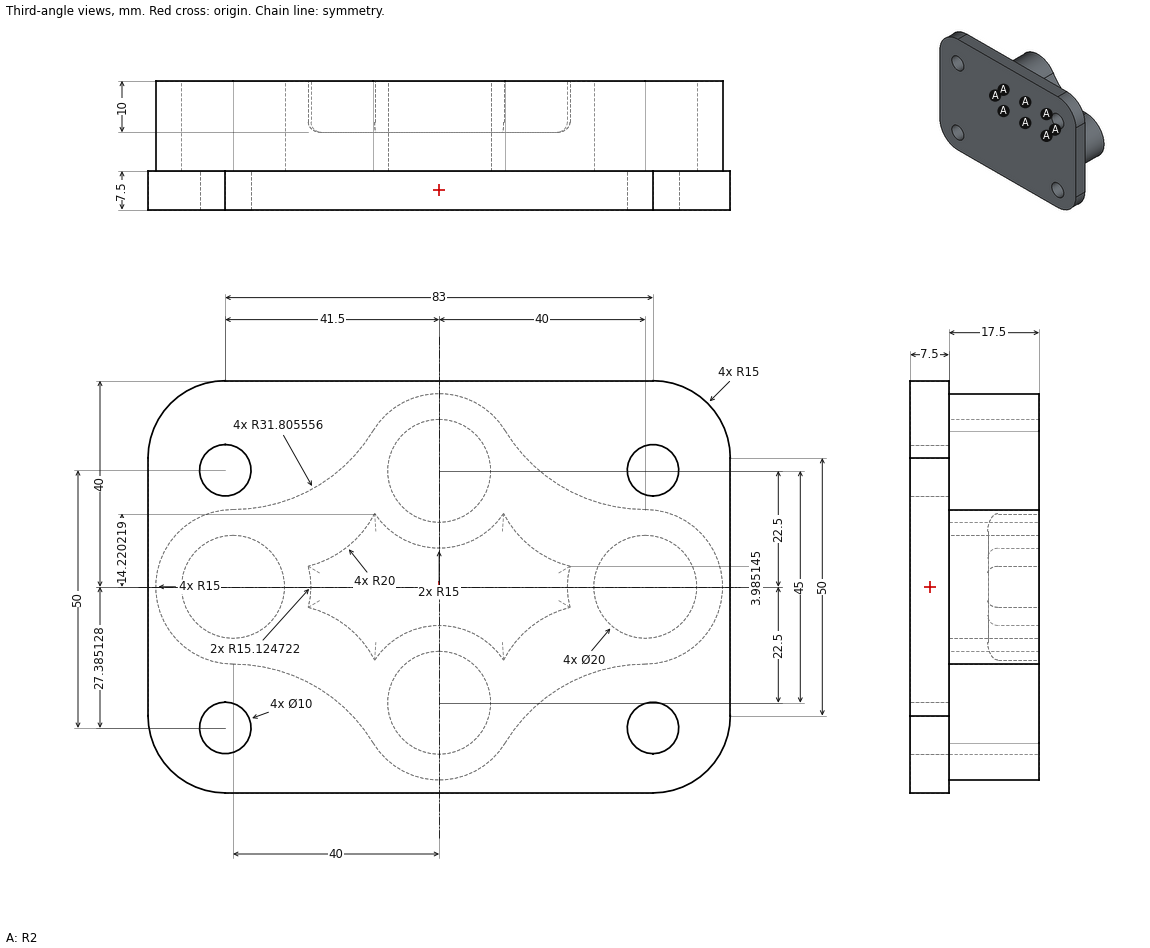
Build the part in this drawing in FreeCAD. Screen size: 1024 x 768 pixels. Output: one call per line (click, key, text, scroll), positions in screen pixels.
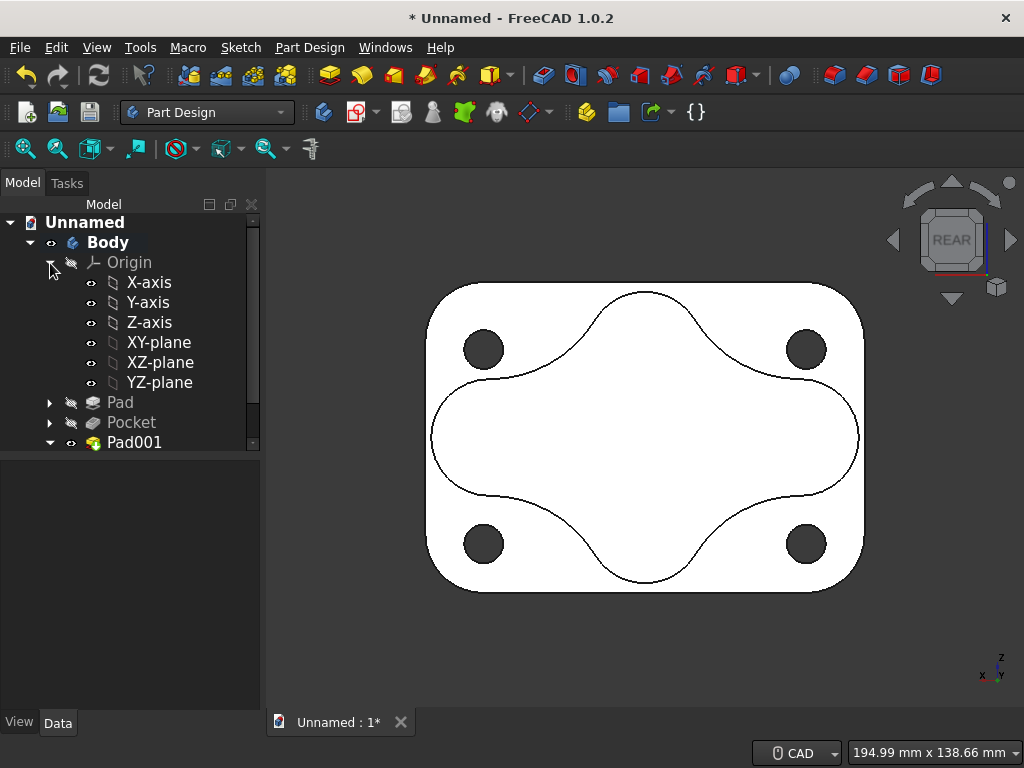
click(136, 363)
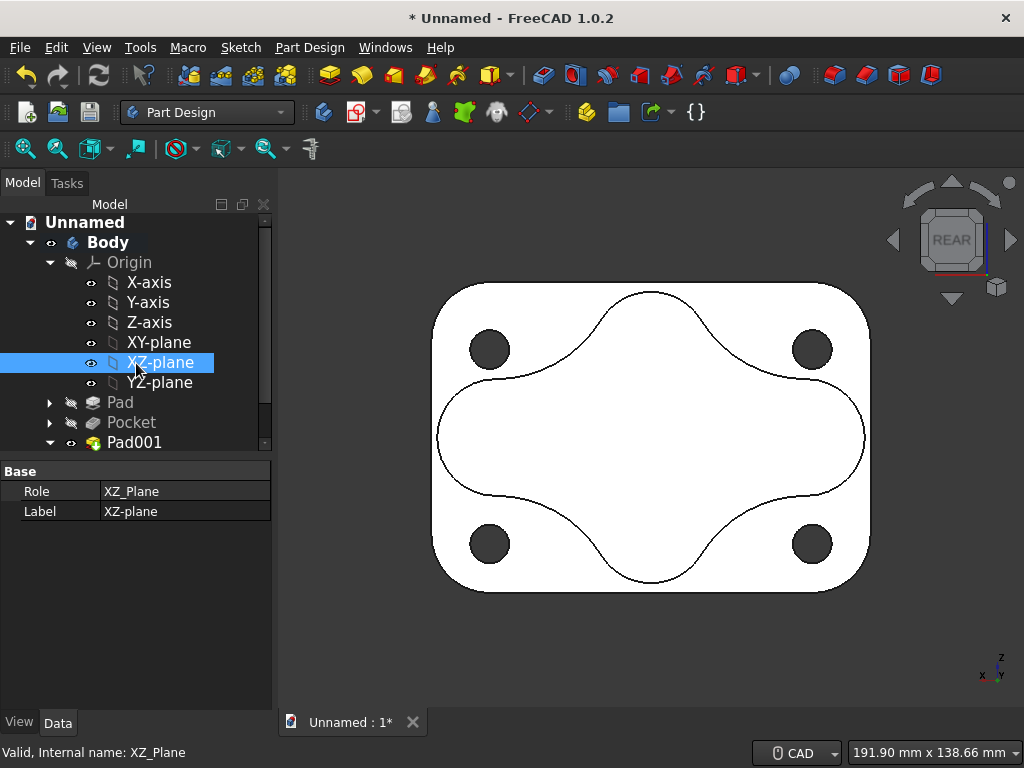
click(530, 112)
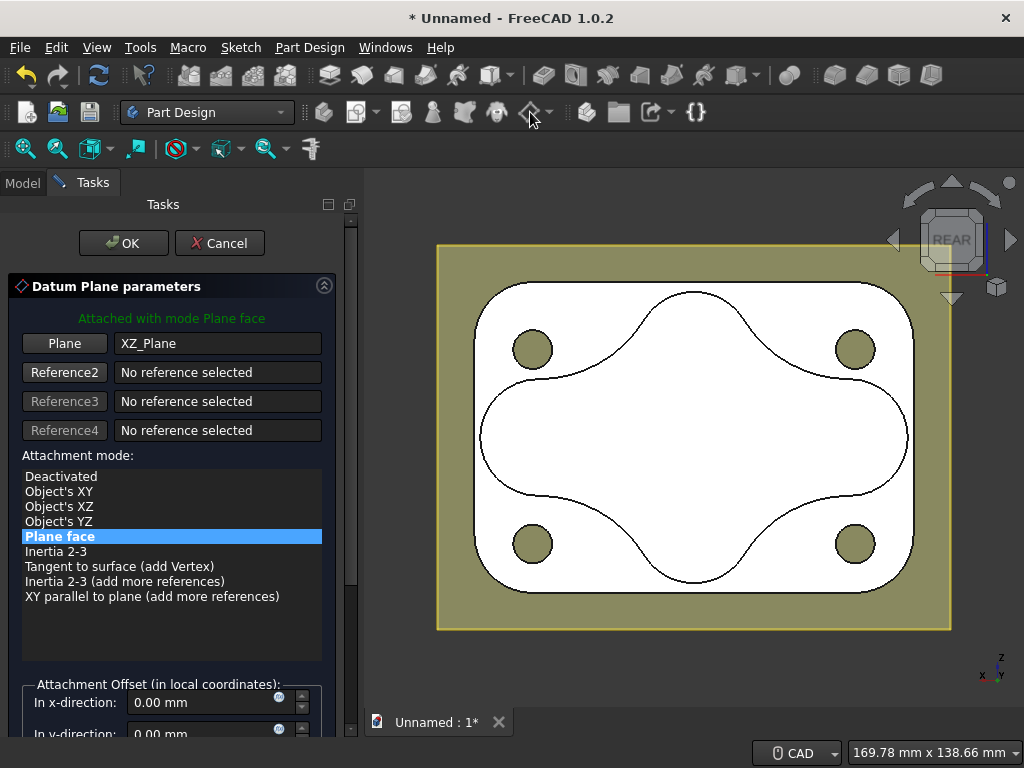
scroll(351, 475, down, 2)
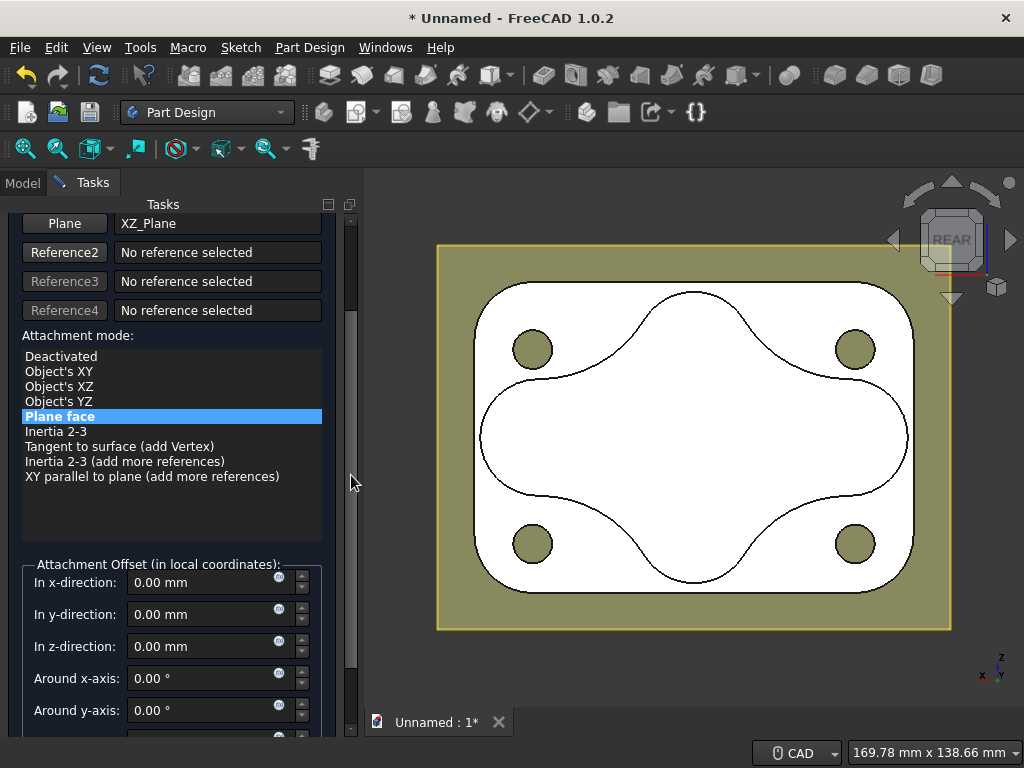
triple_click(210, 646)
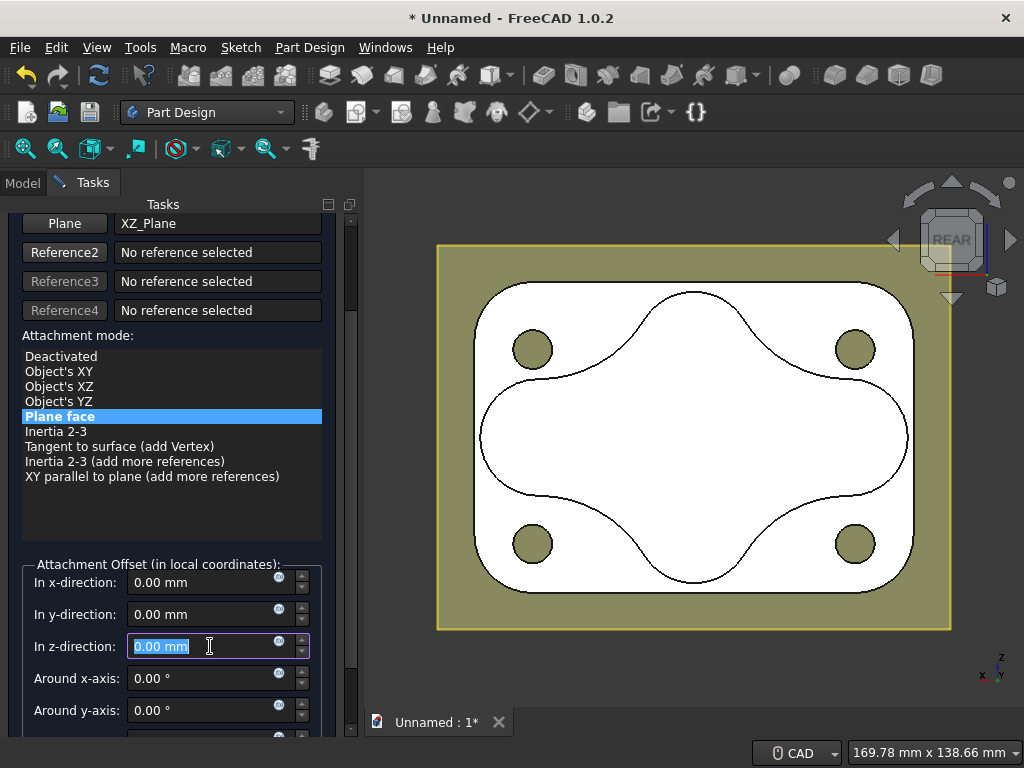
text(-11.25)
key(Tab)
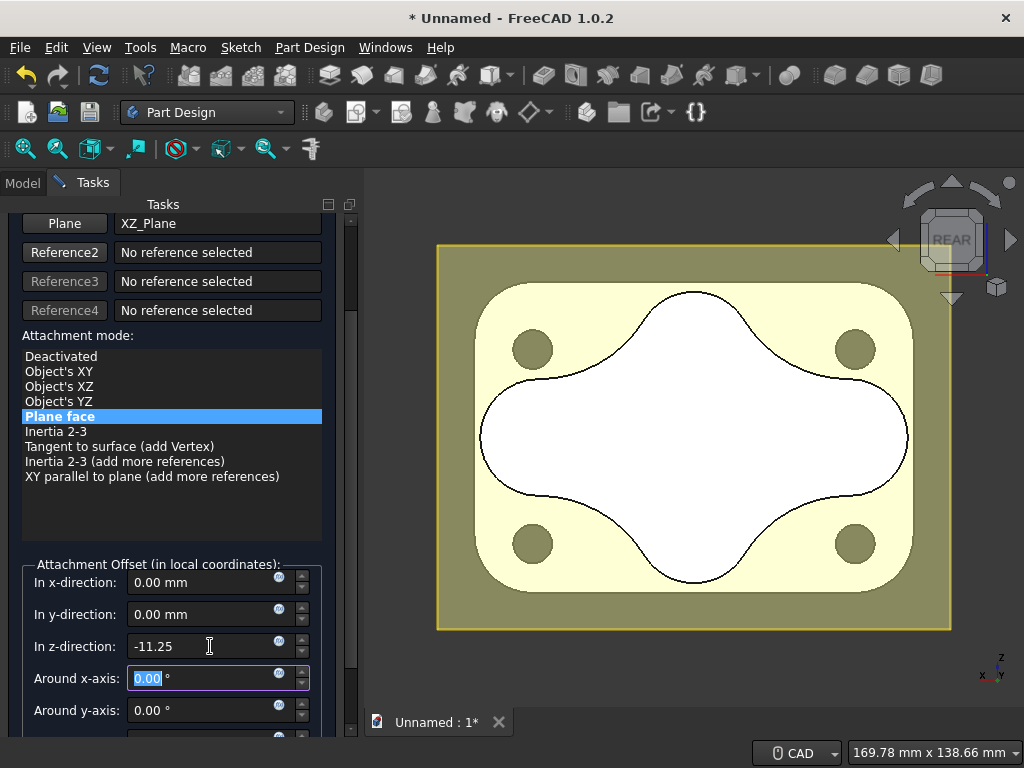
scroll(351, 475, up, 3)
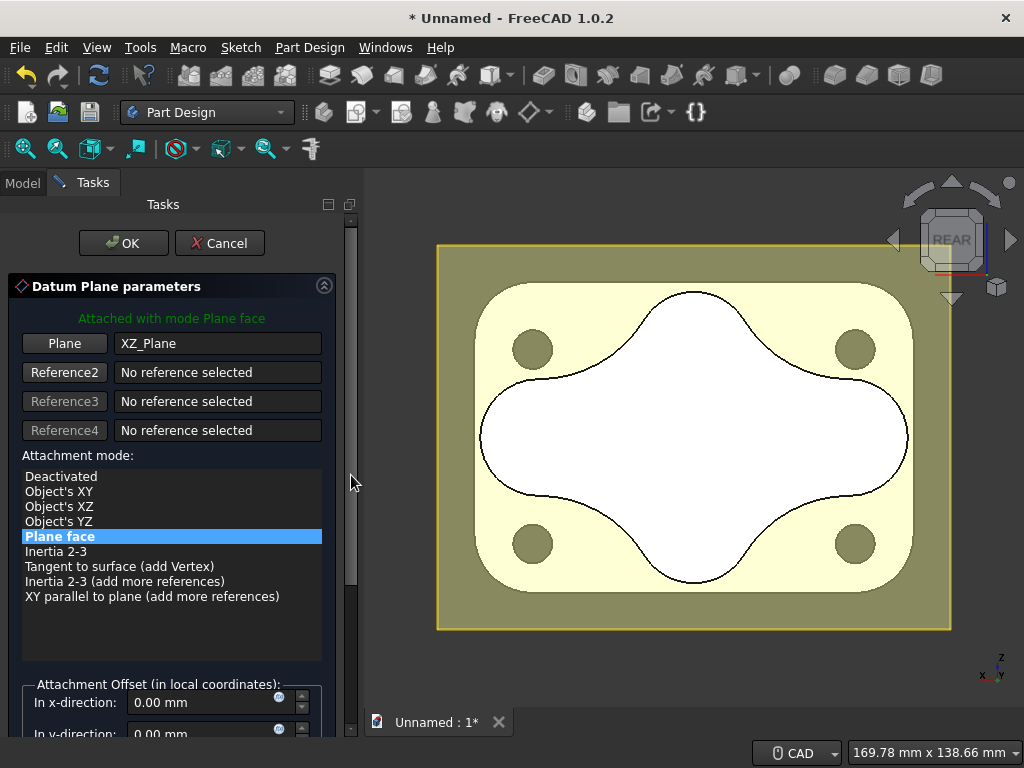
click(124, 243)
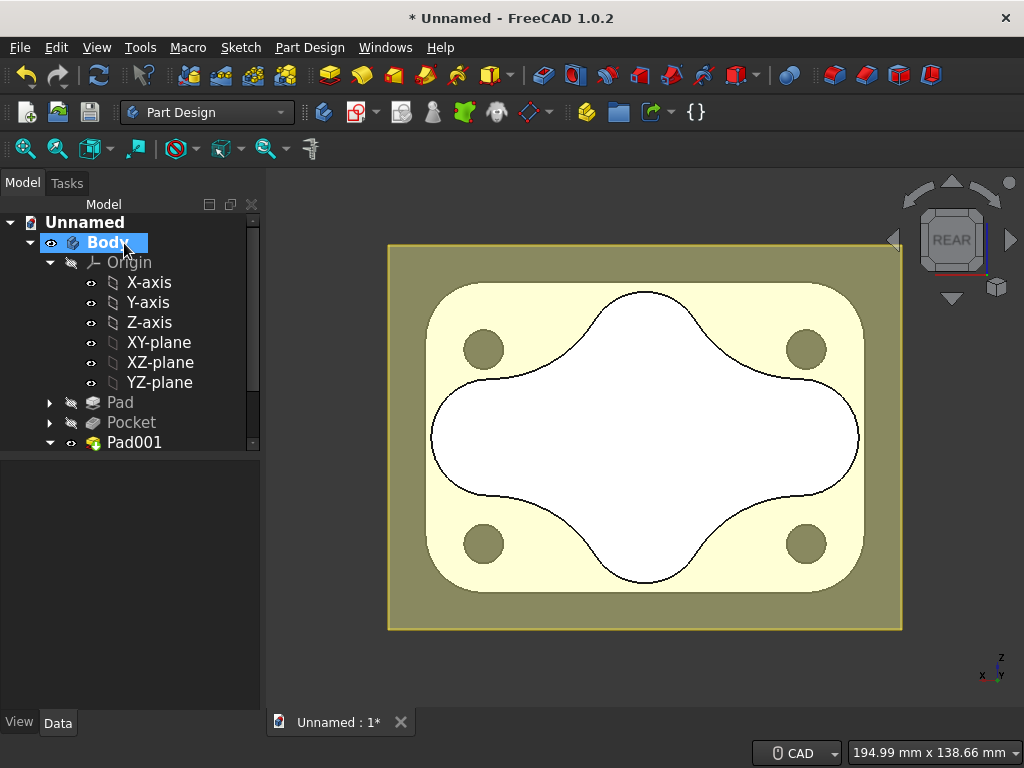
scroll(100, 338, down, 3)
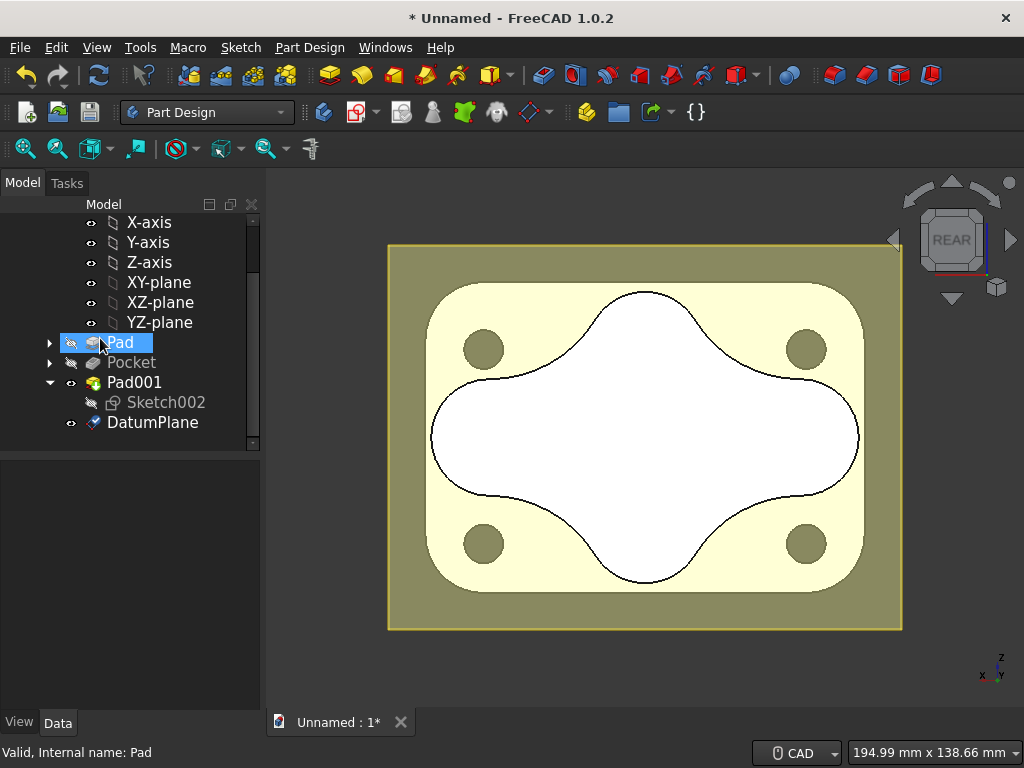
click(116, 423)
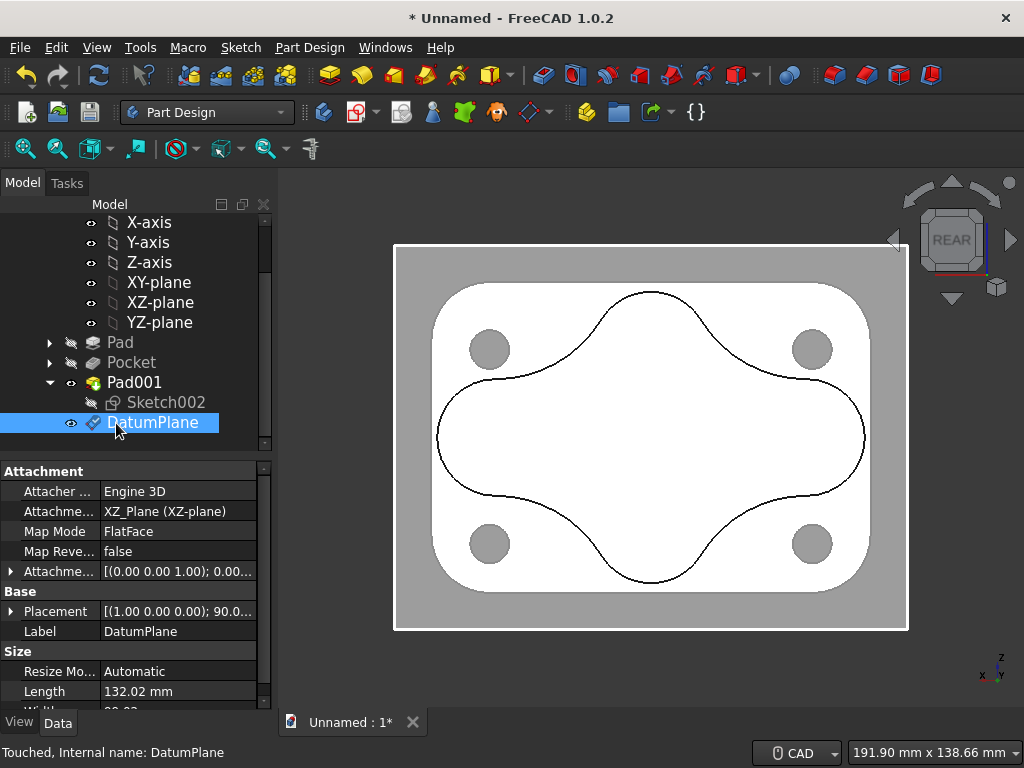
click(356, 112)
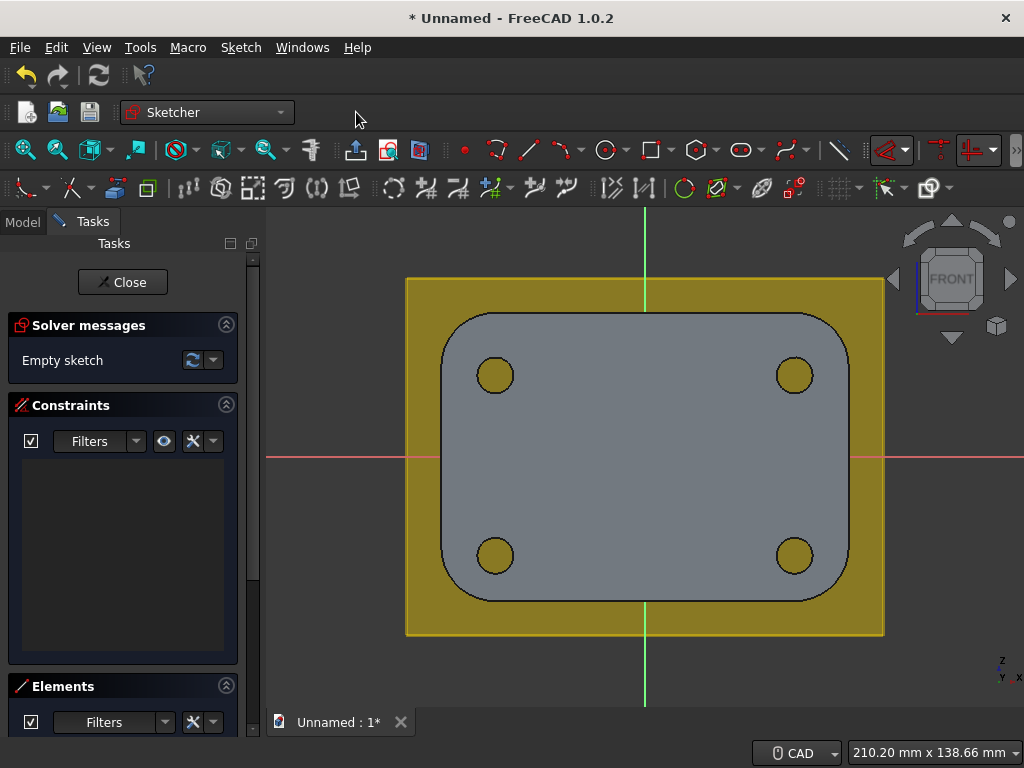
click(420, 150)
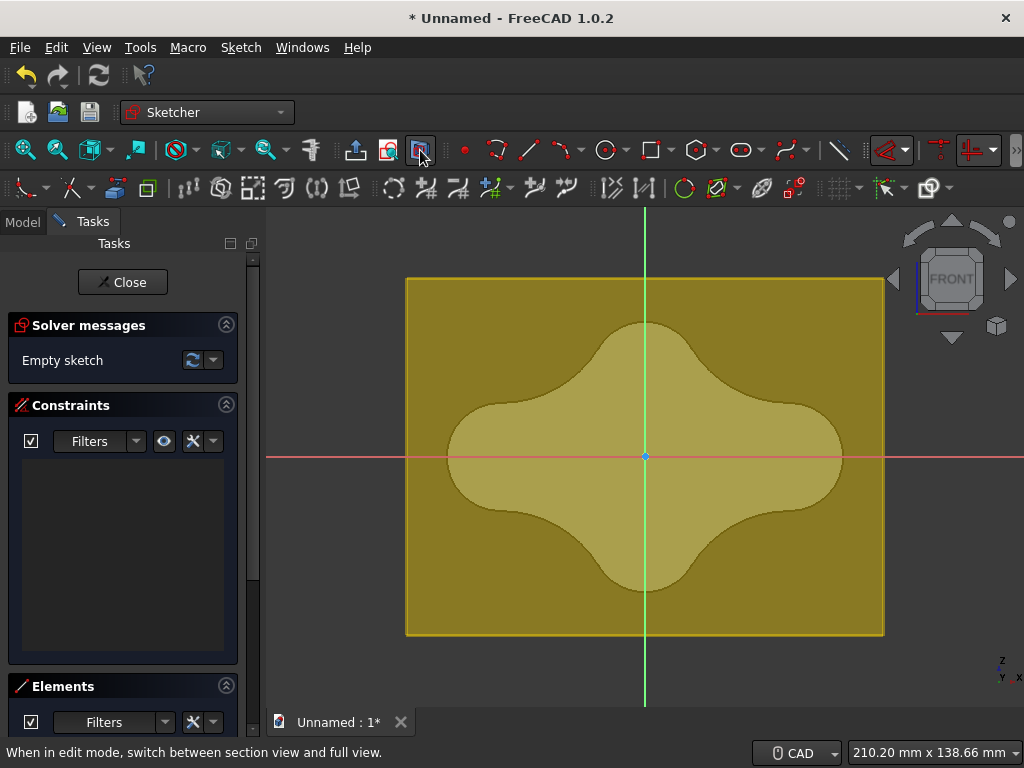
scroll(701, 457, up, 4)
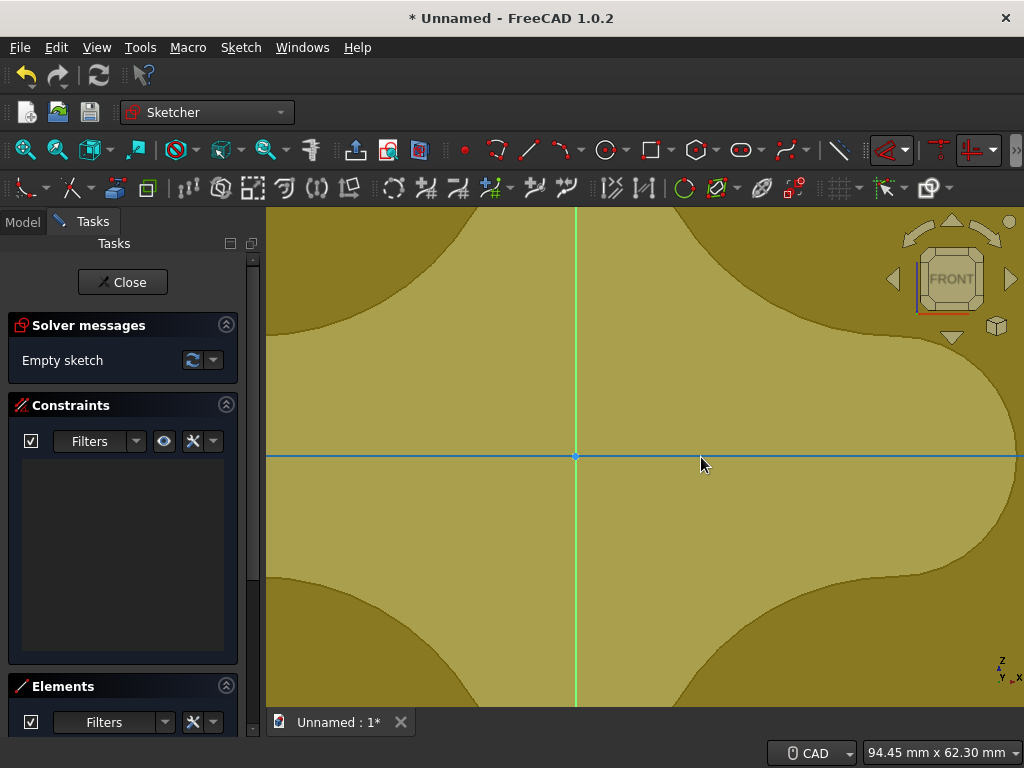
click(562, 150)